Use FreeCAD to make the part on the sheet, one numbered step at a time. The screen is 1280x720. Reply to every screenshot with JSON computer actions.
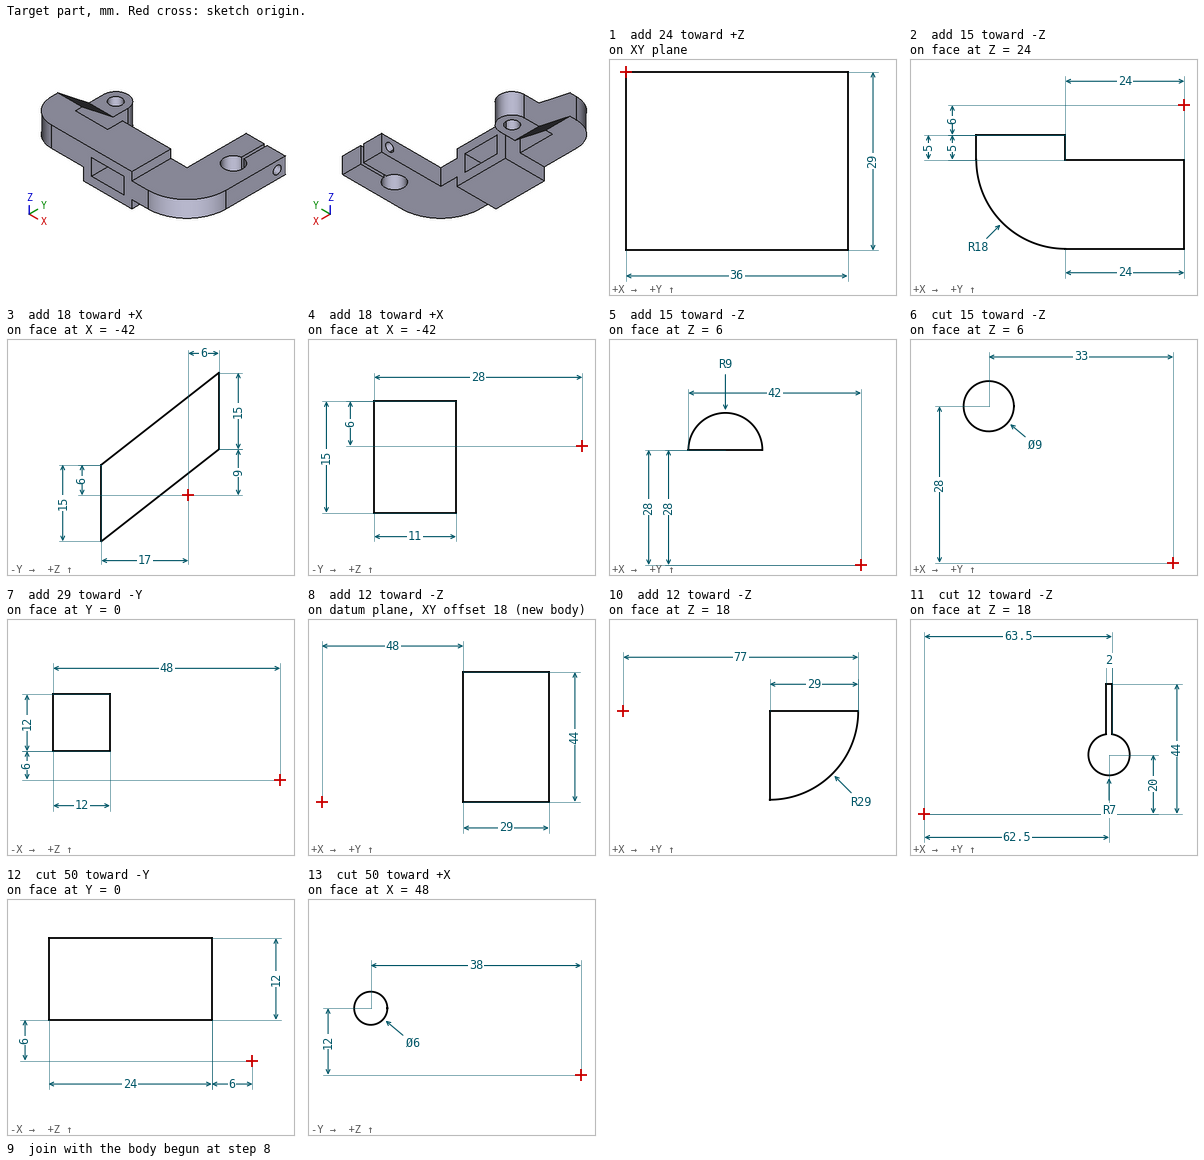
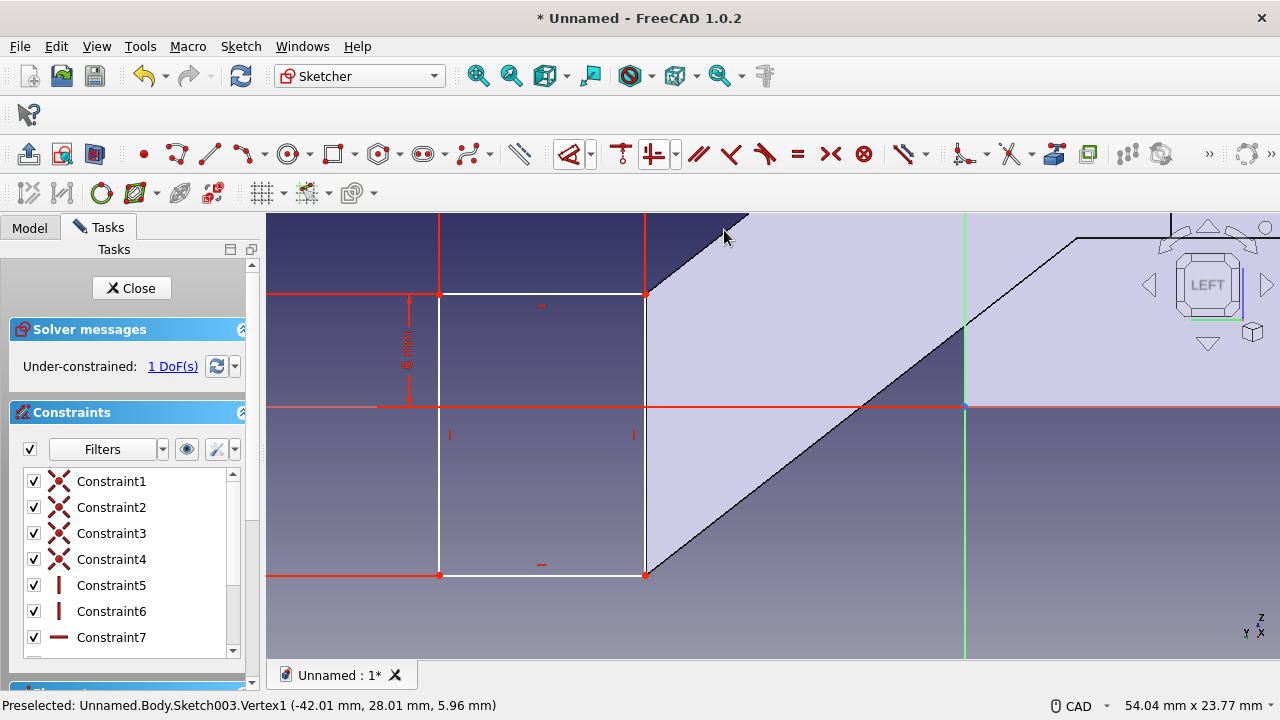
{"action": "left_click", "coordinate": [439, 294]}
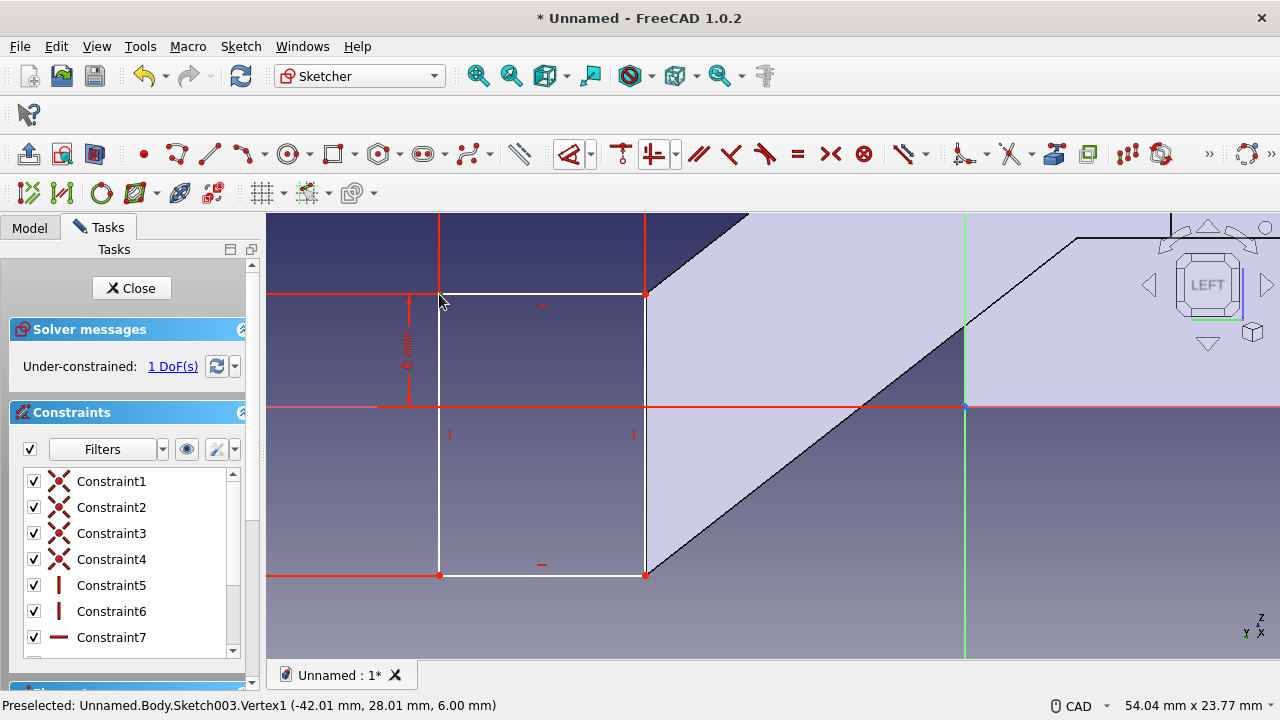
{"action": "left_click", "coordinate": [590, 154]}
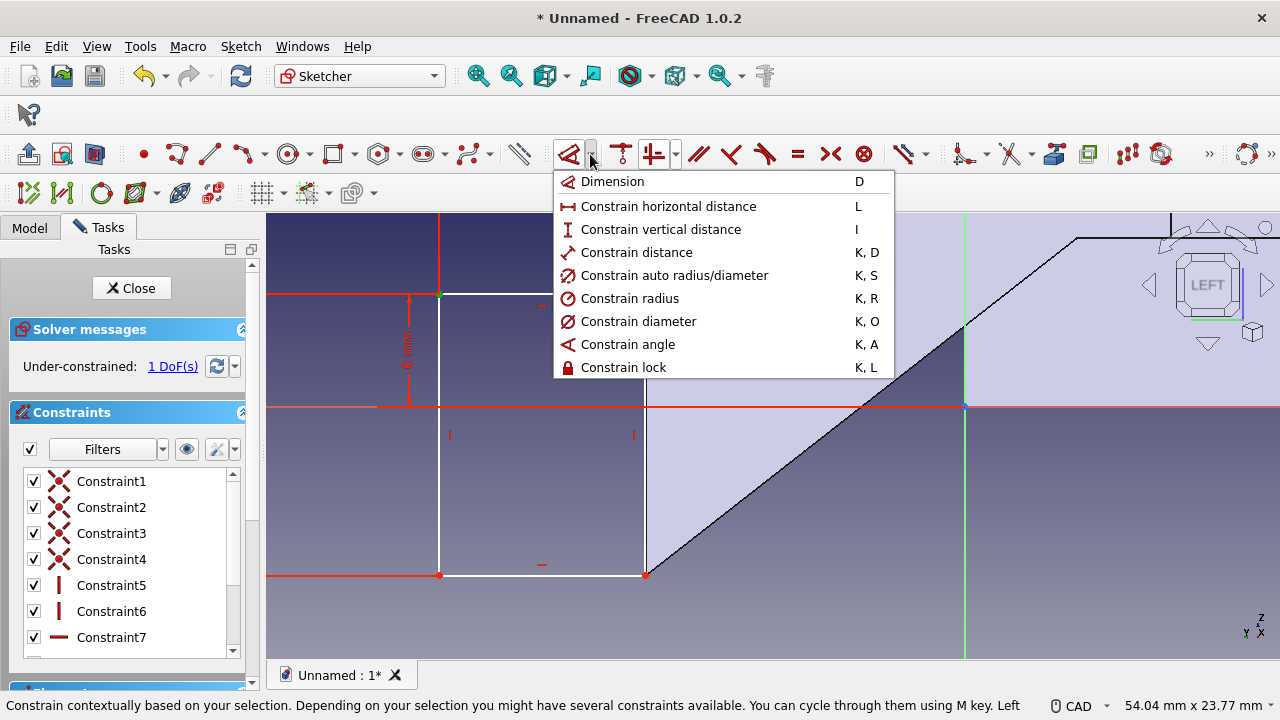
{"action": "left_click", "coordinate": [724, 206]}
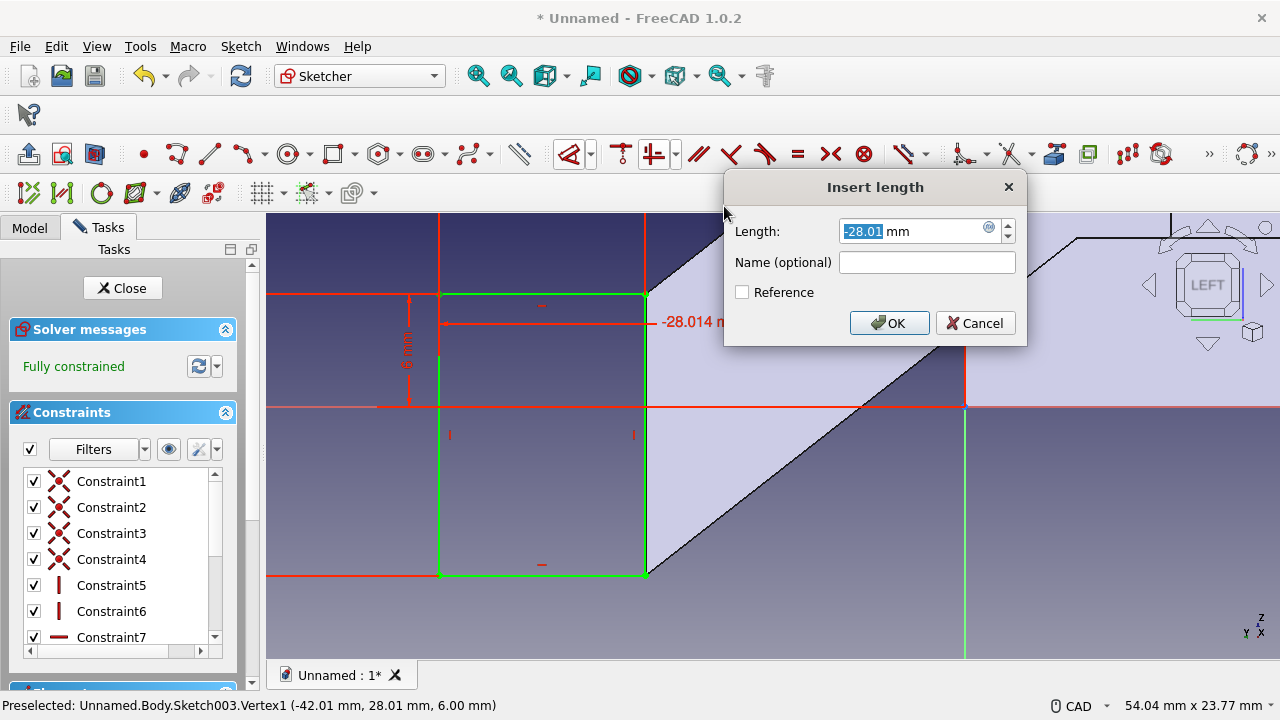
{"action": "type", "text": "-28"}
{"action": "key", "text": "Return"}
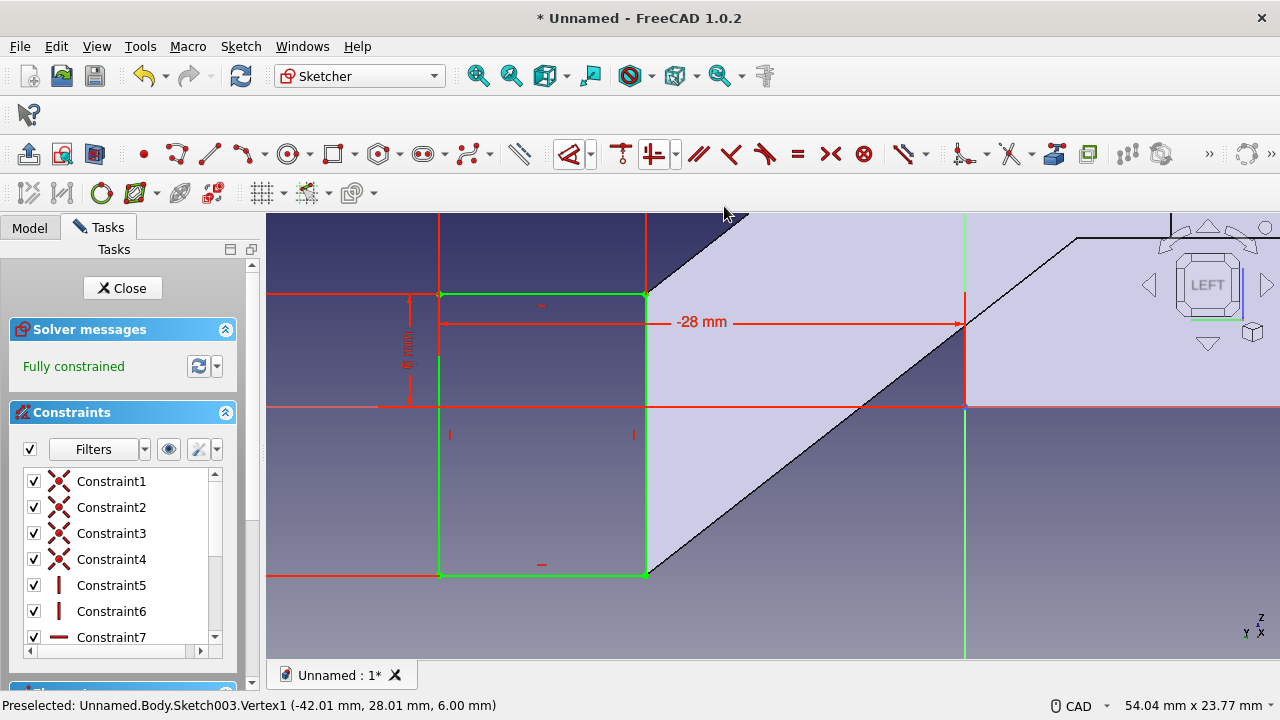
{"action": "left_click", "coordinate": [123, 288]}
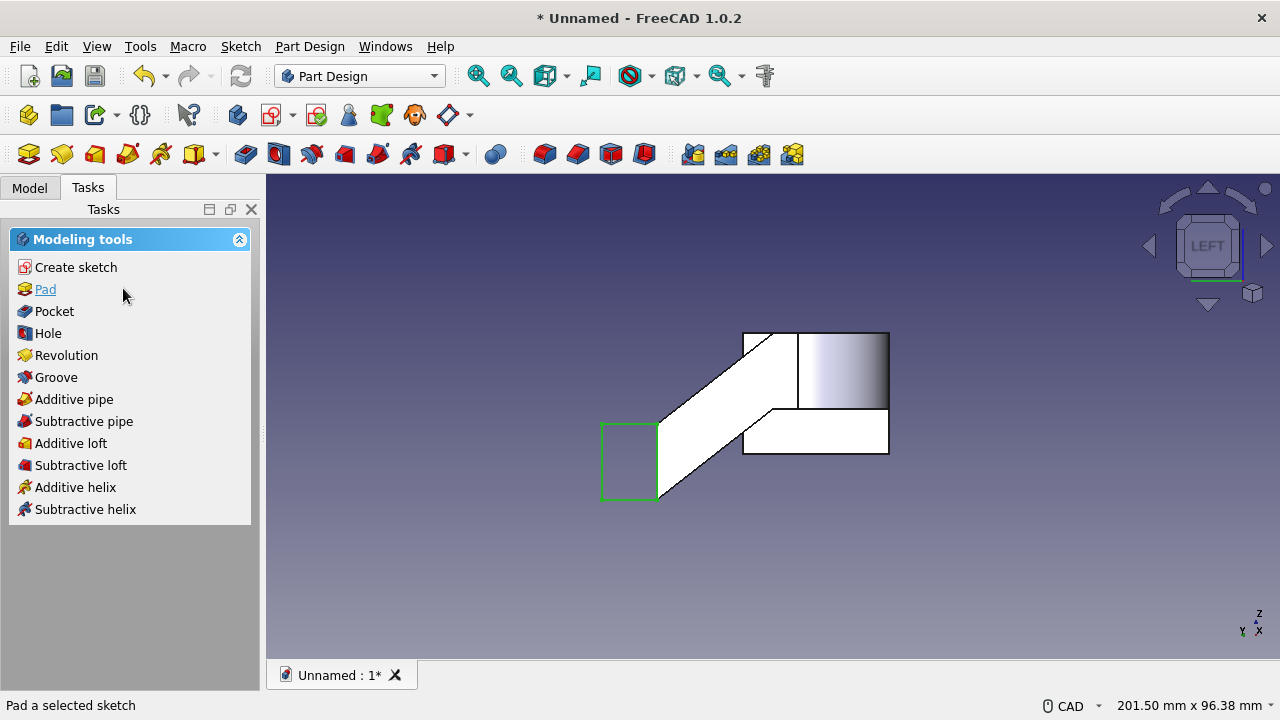
{"action": "left_click", "coordinate": [29, 154]}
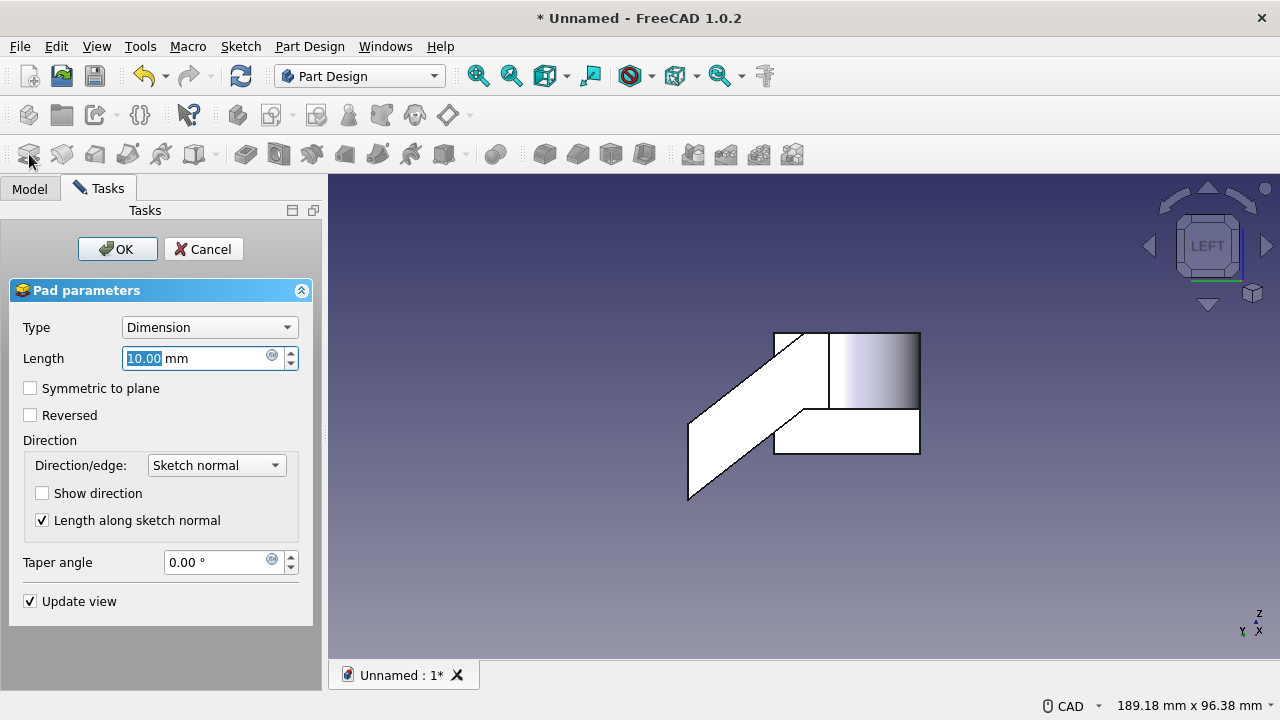
{"action": "type", "text": "18"}
{"action": "key", "text": "Tab"}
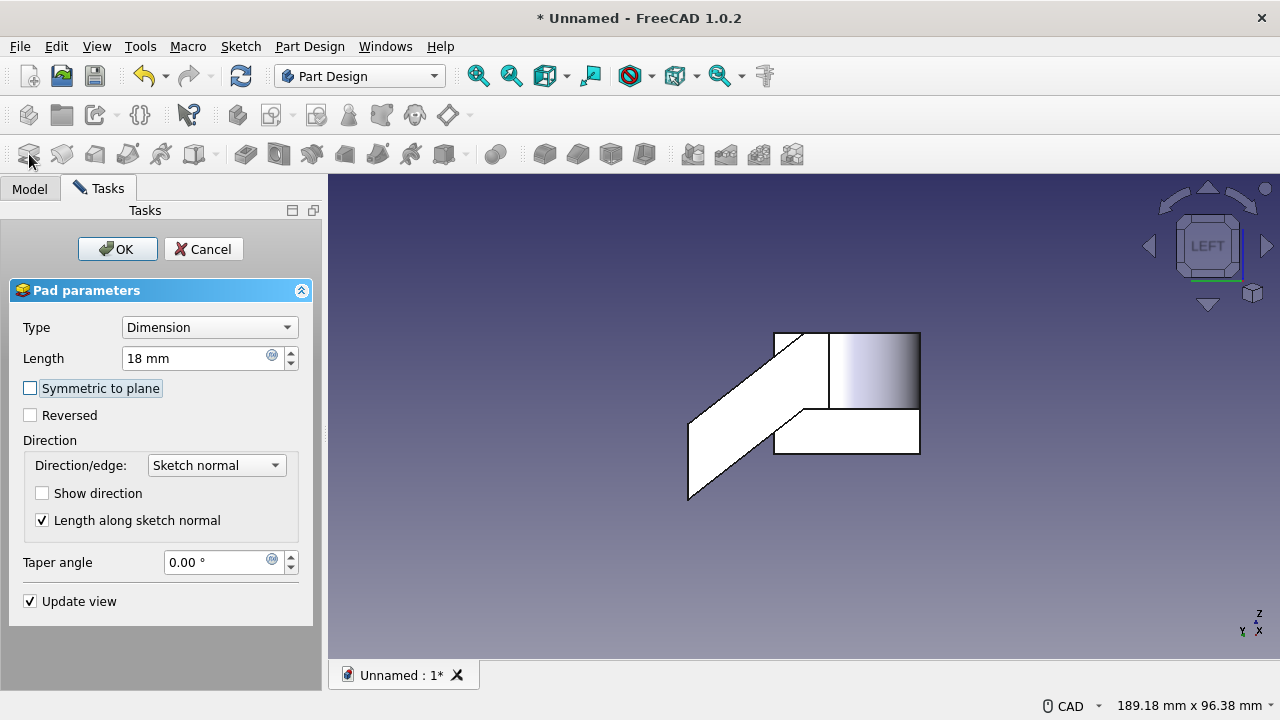
{"action": "left_click", "coordinate": [31, 415]}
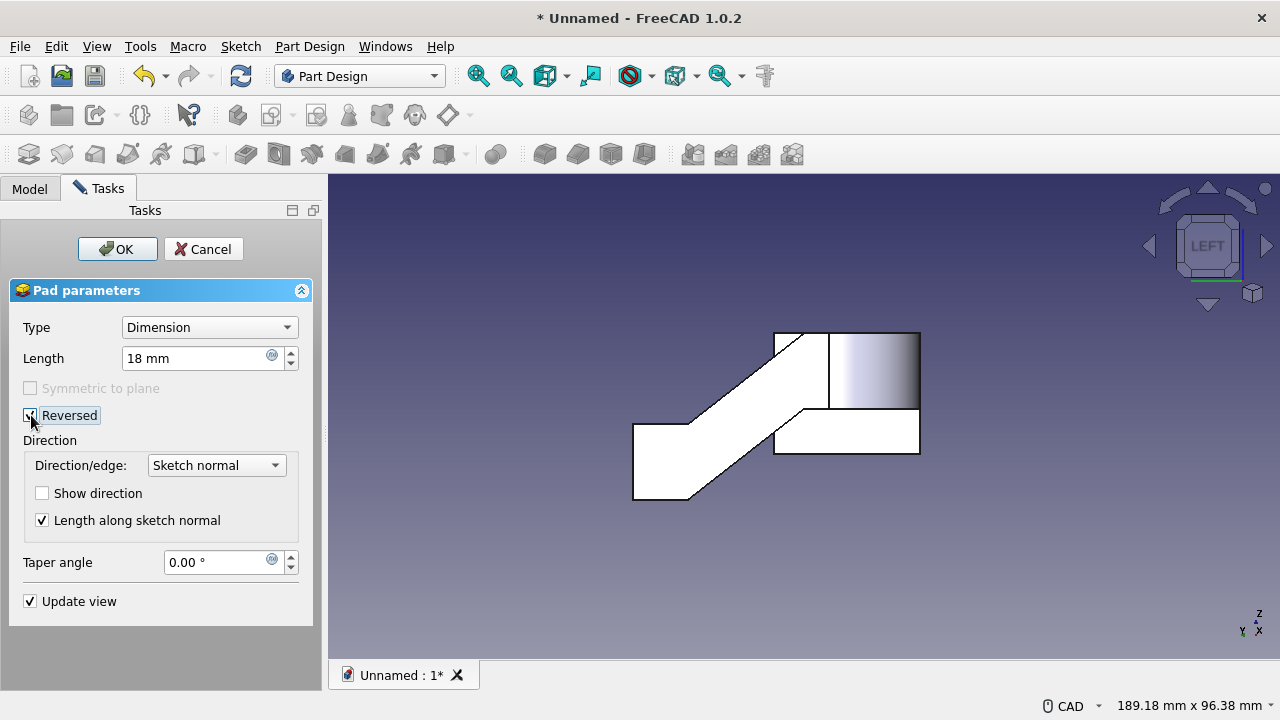
{"action": "left_click", "coordinate": [118, 249]}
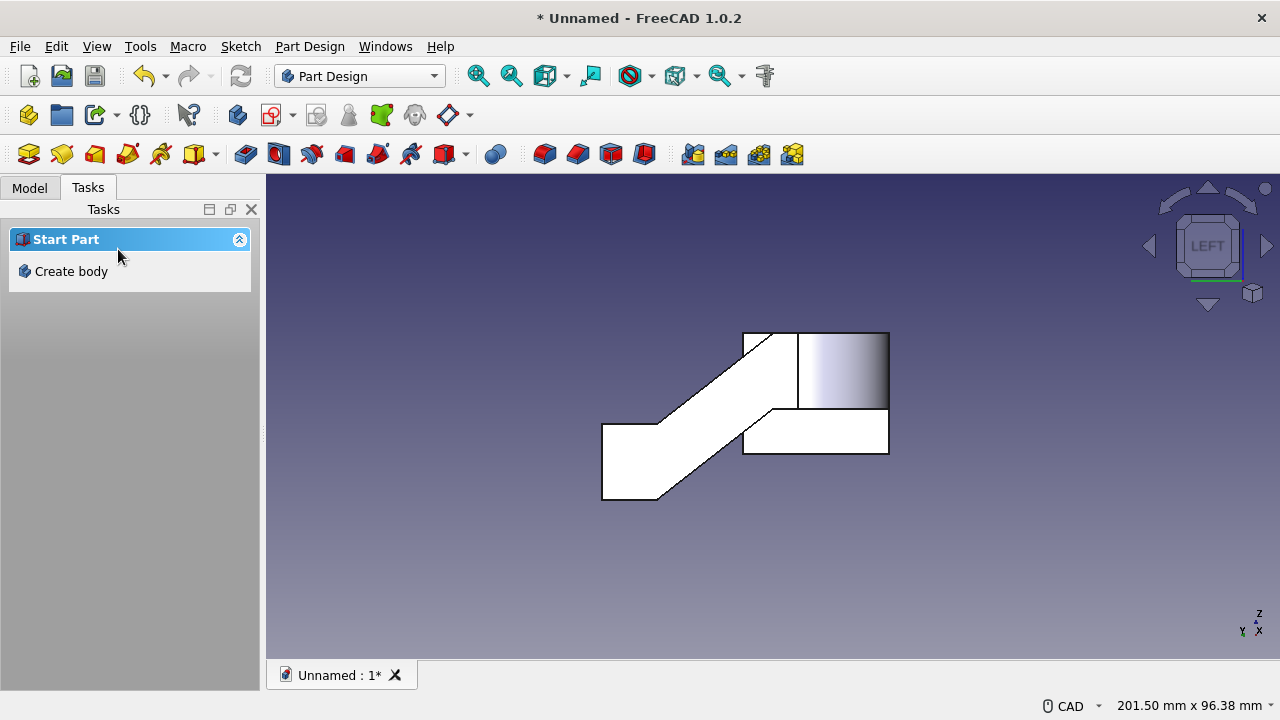
{"action": "left_click", "coordinate": [479, 76]}